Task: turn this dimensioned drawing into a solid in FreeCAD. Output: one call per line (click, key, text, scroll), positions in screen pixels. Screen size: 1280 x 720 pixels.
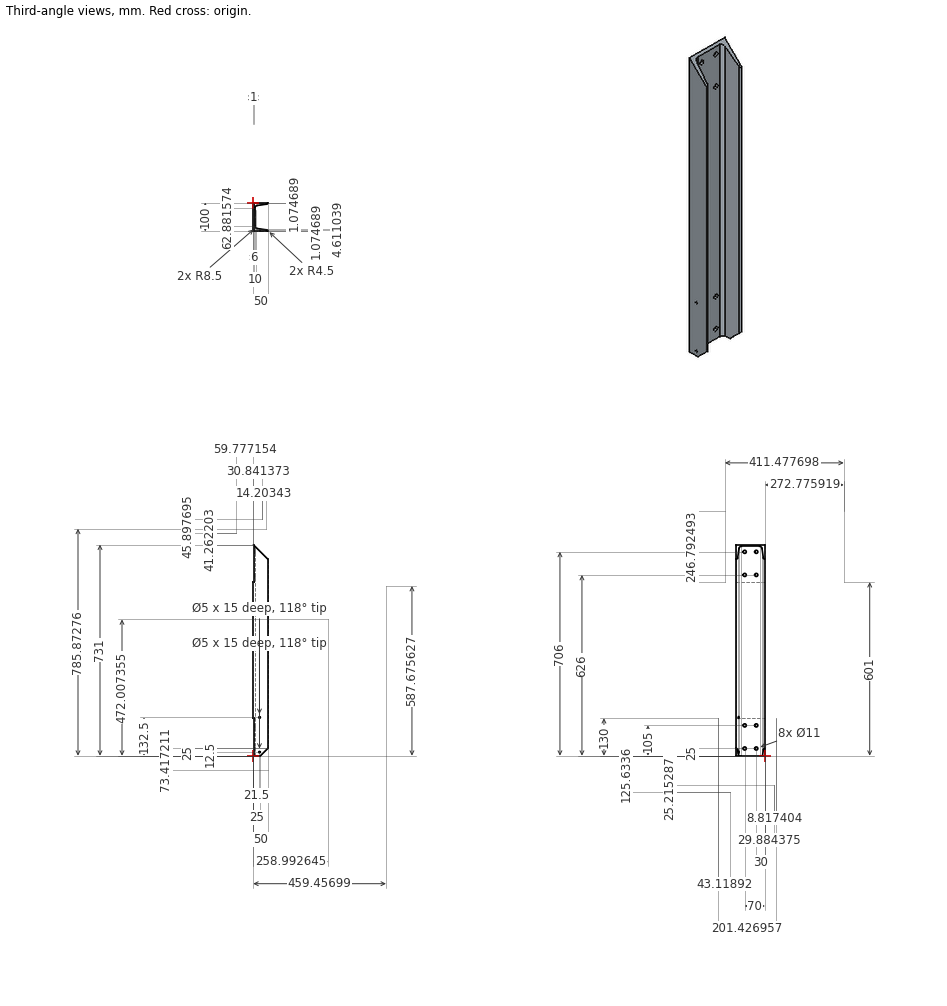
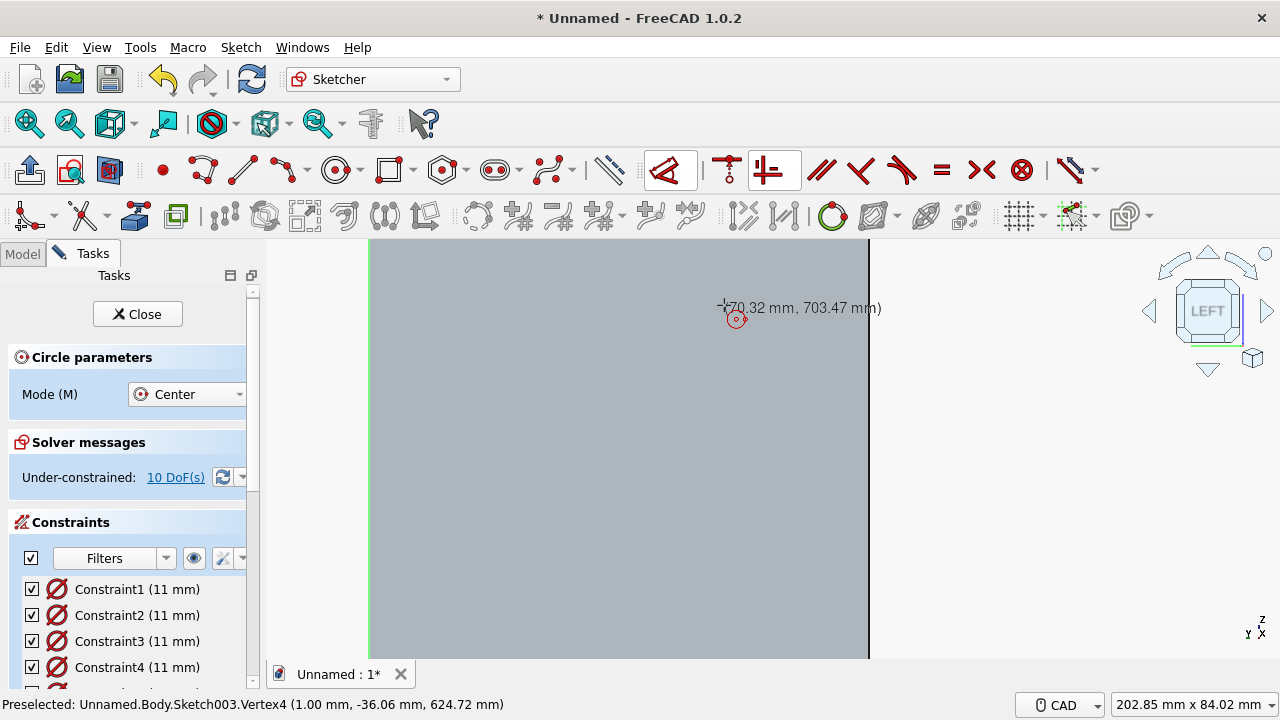
scroll(716, 320, down, 13)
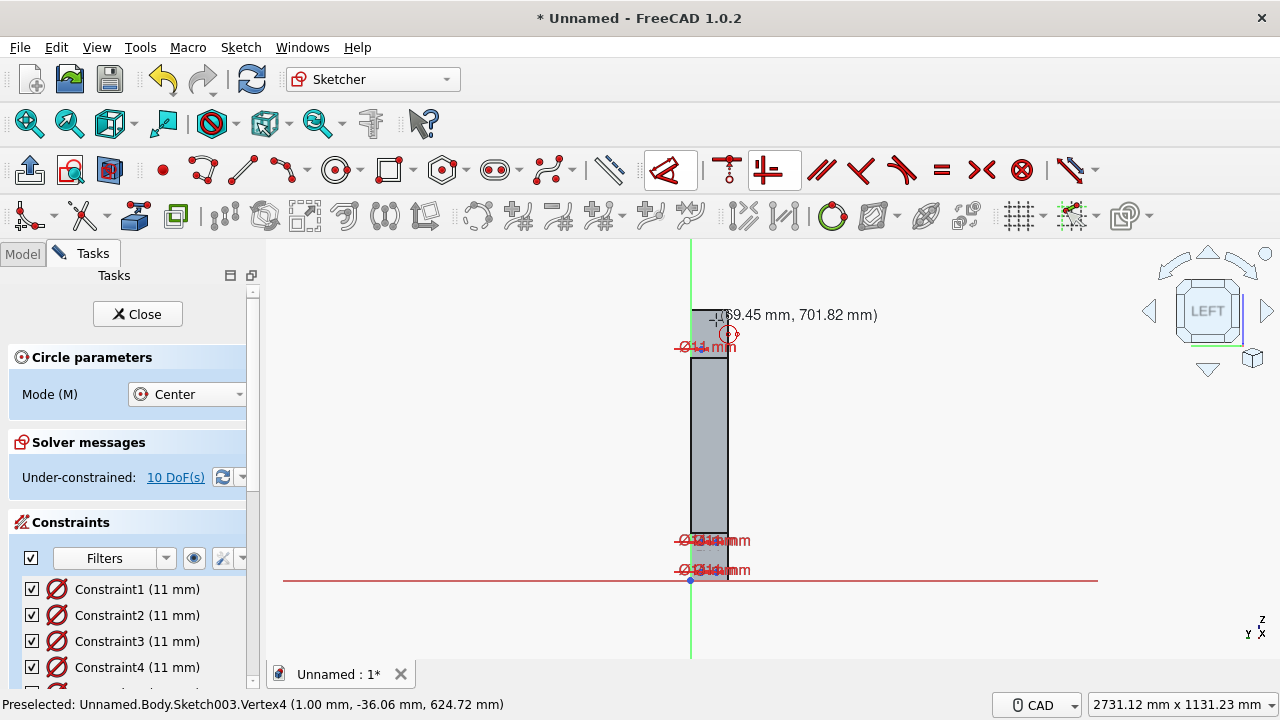
click(717, 319)
move(718, 317)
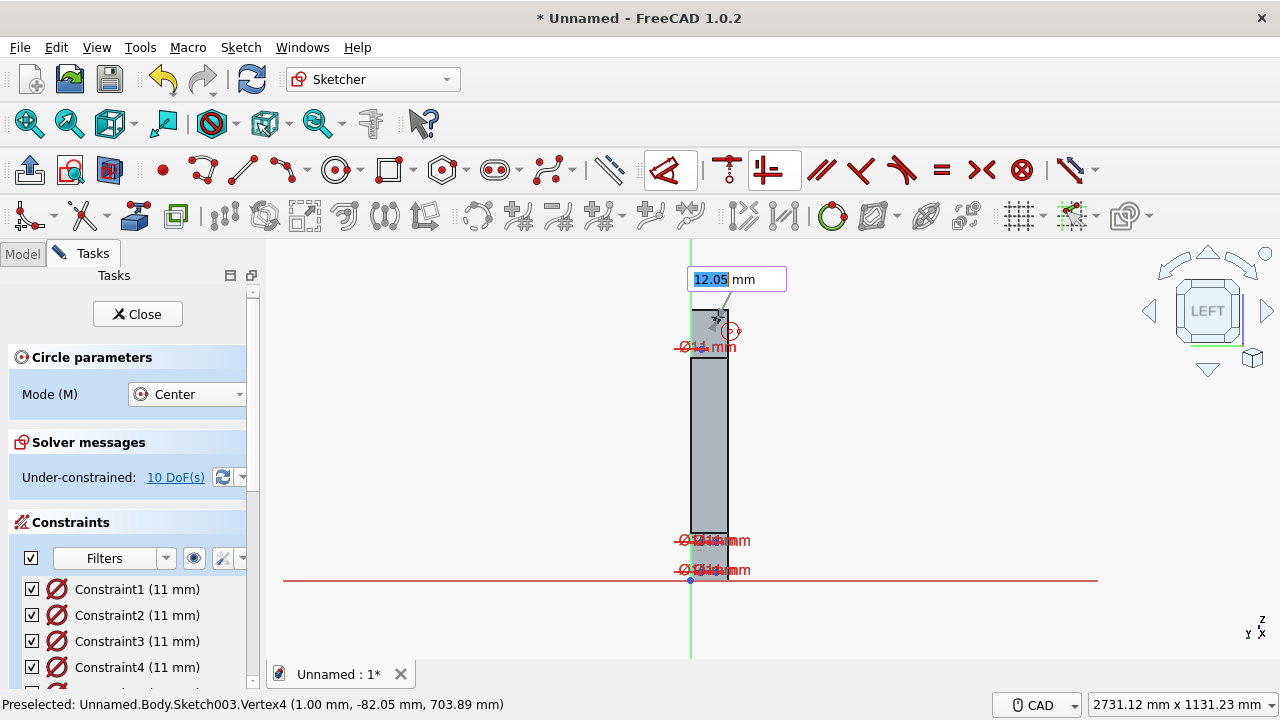
text(11)
key(Return)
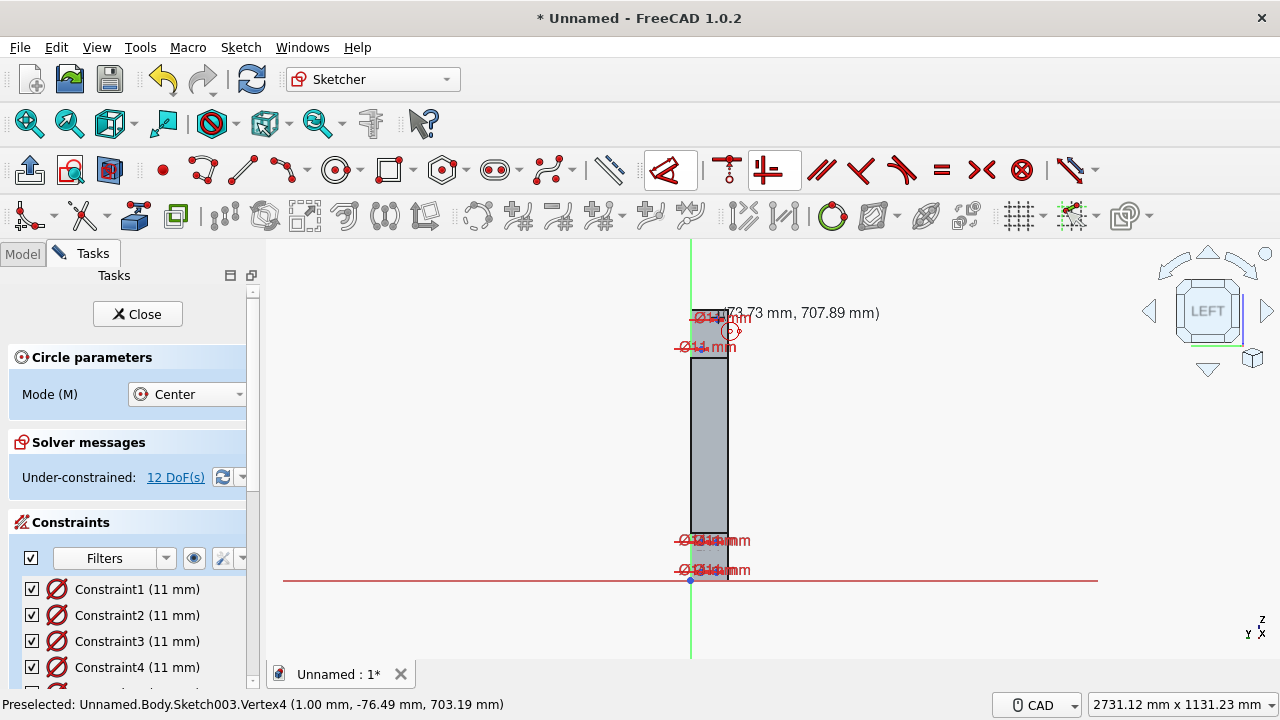
scroll(717, 348, up, 13)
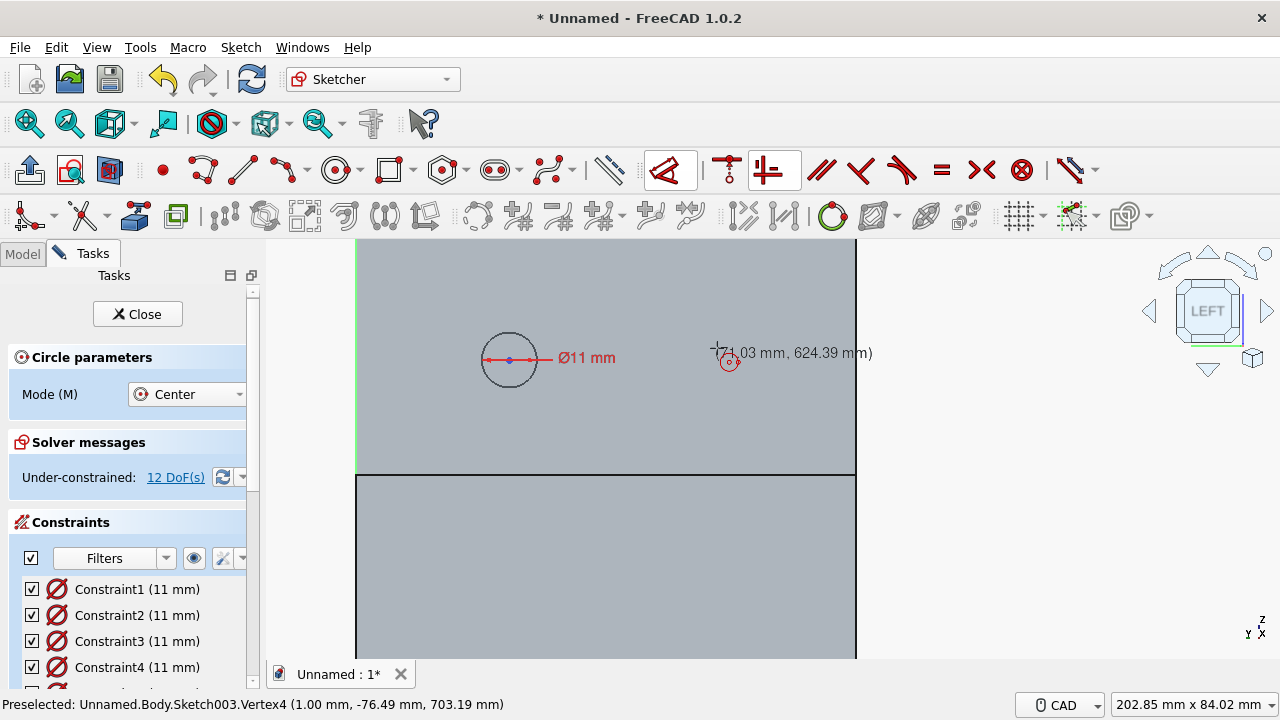
scroll(717, 349, down, 13)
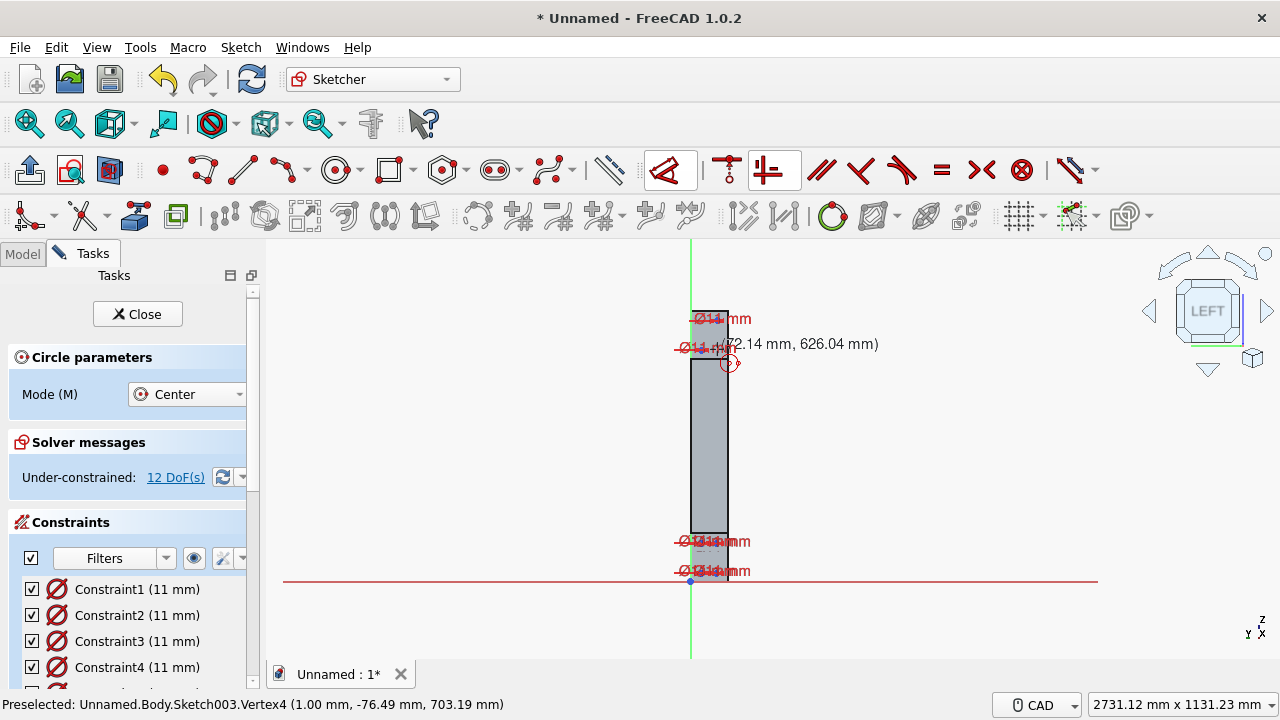
scroll(717, 349, up, 2)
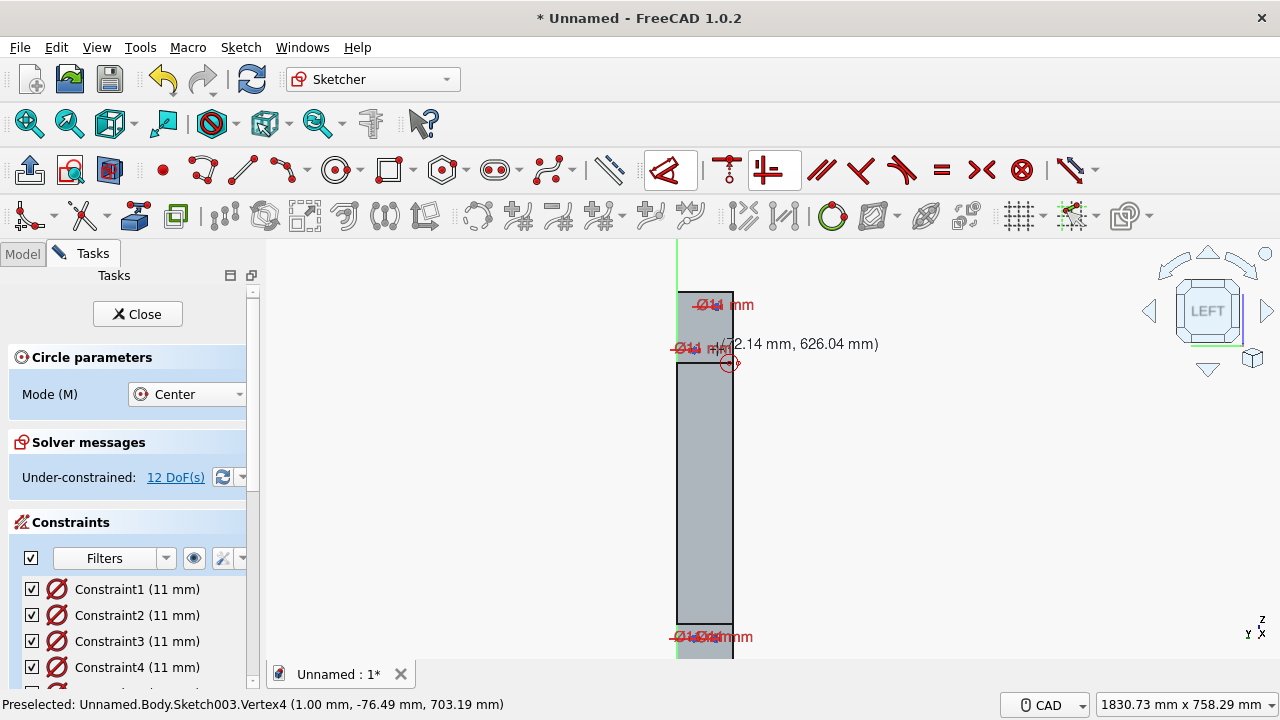
click(716, 349)
move(718, 347)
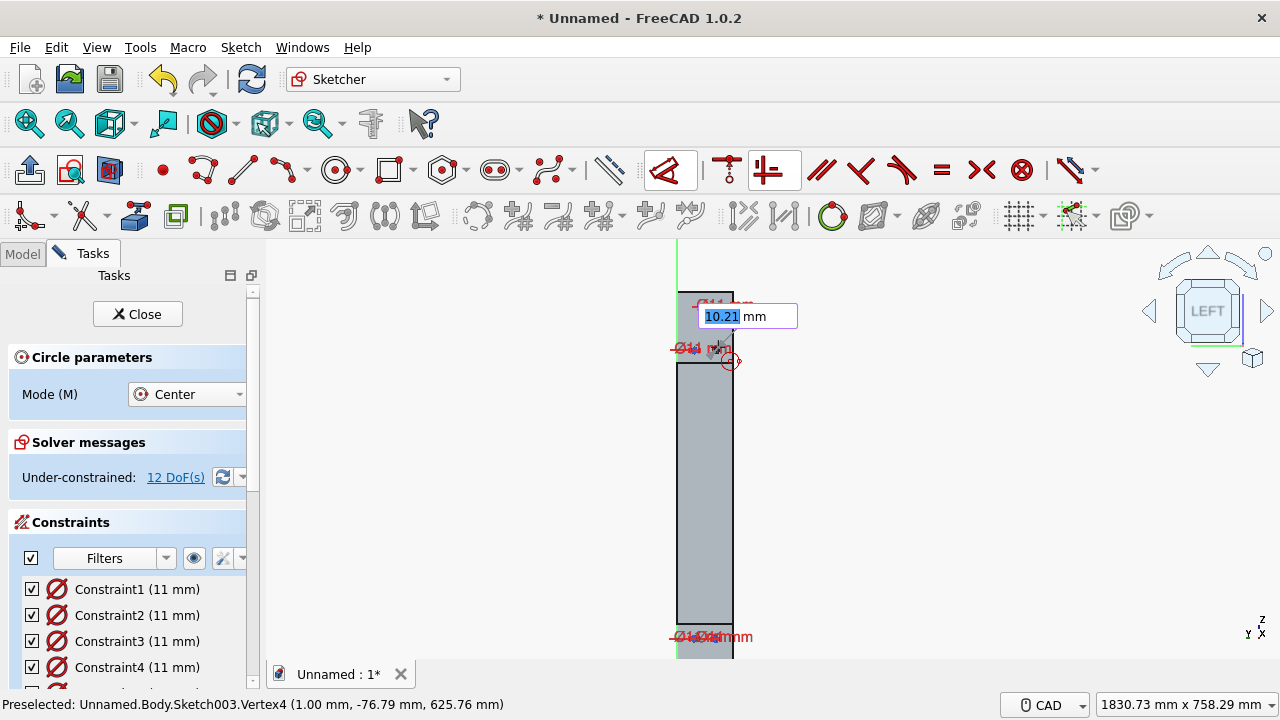
text(11)
key(Return)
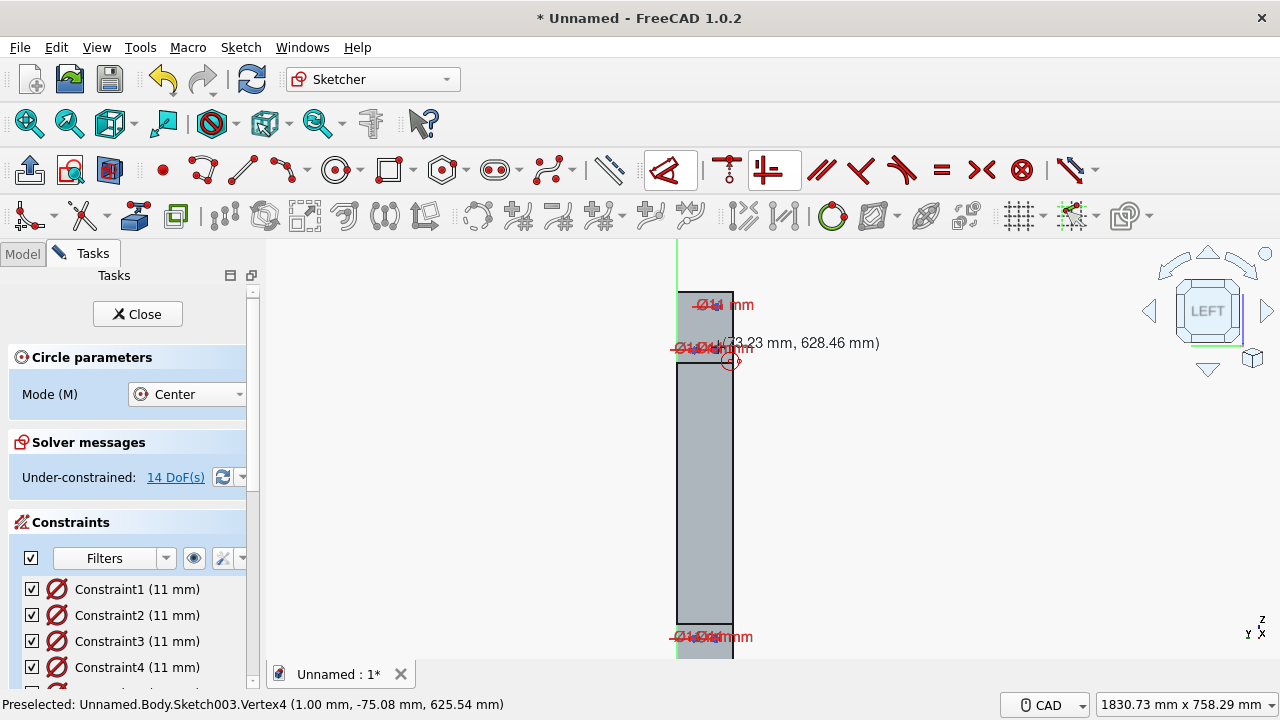
scroll(694, 305, up, 11)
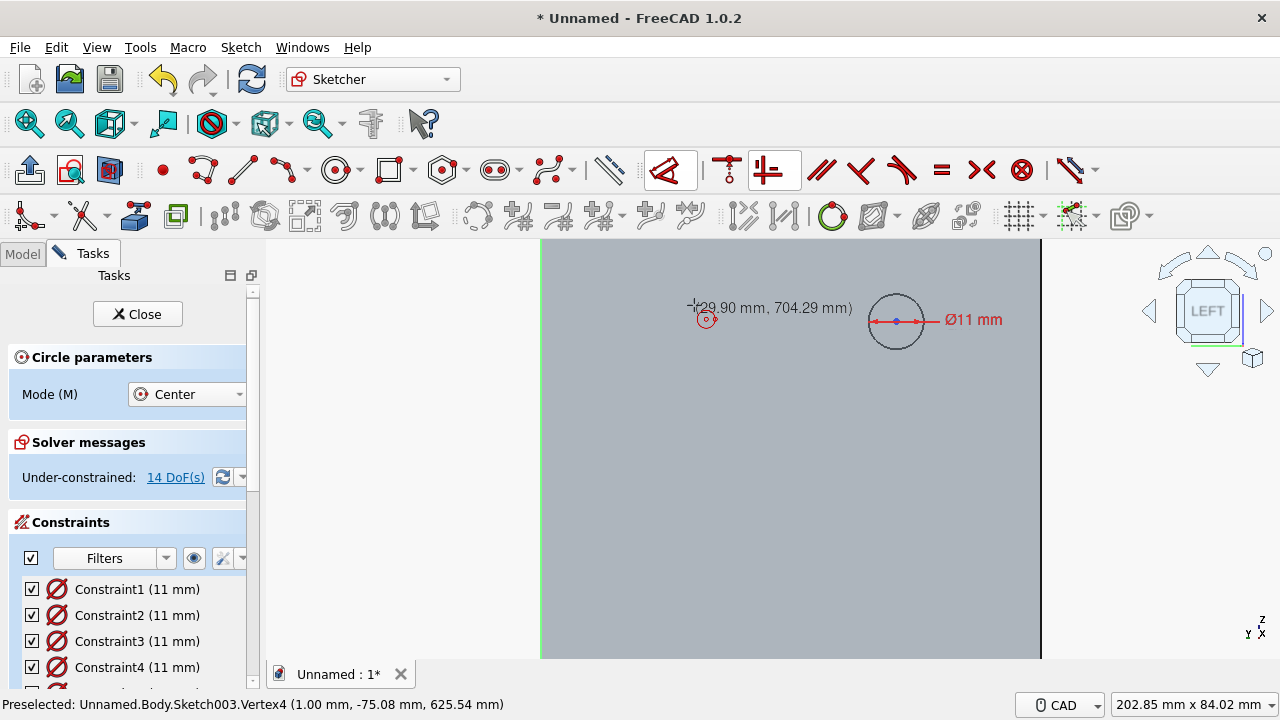
scroll(702, 320, down, 13)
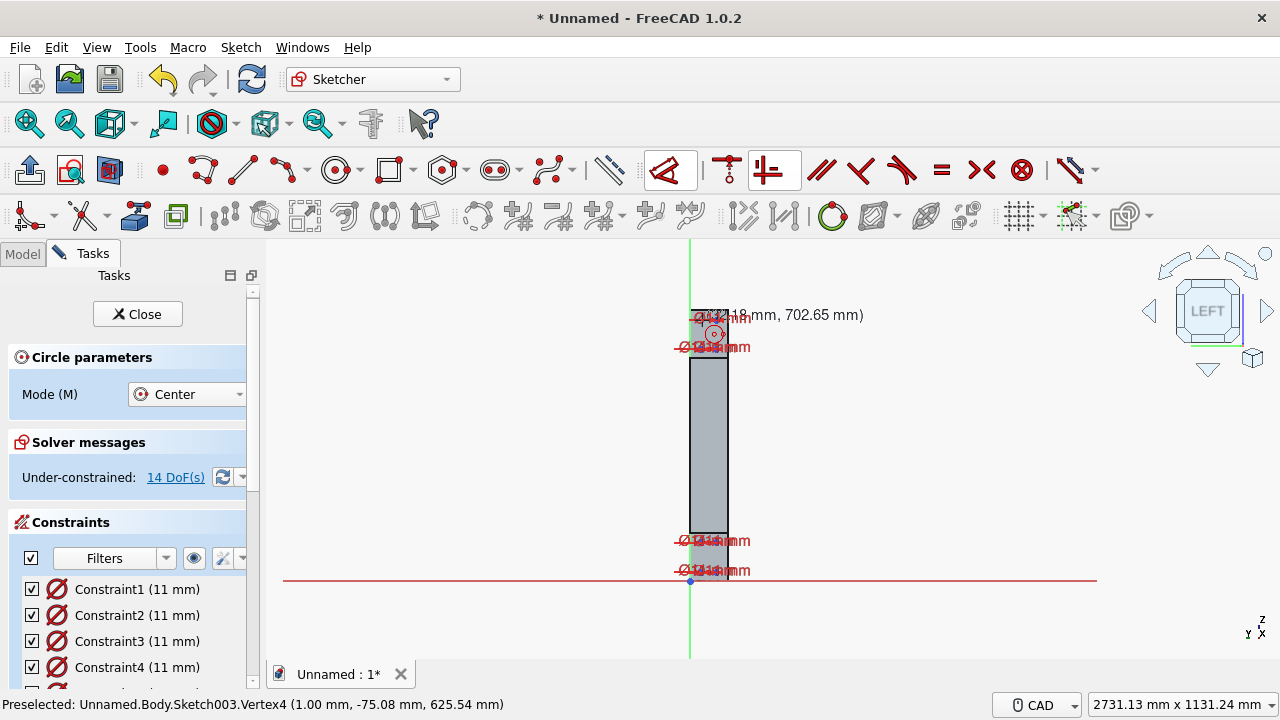
scroll(702, 319, up, 2)